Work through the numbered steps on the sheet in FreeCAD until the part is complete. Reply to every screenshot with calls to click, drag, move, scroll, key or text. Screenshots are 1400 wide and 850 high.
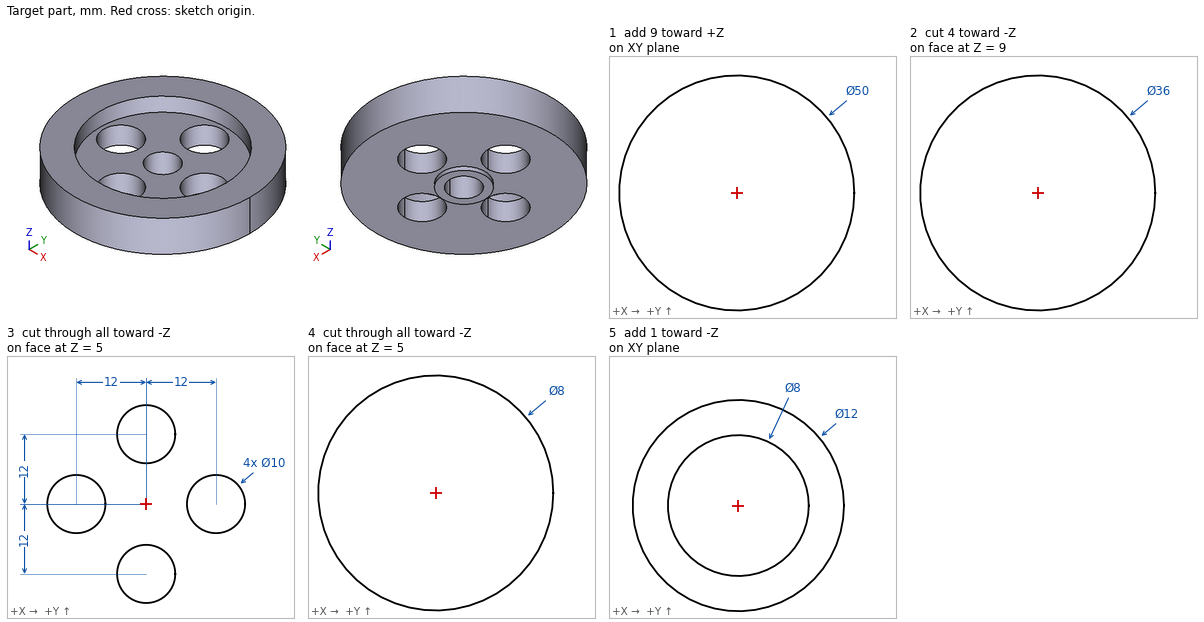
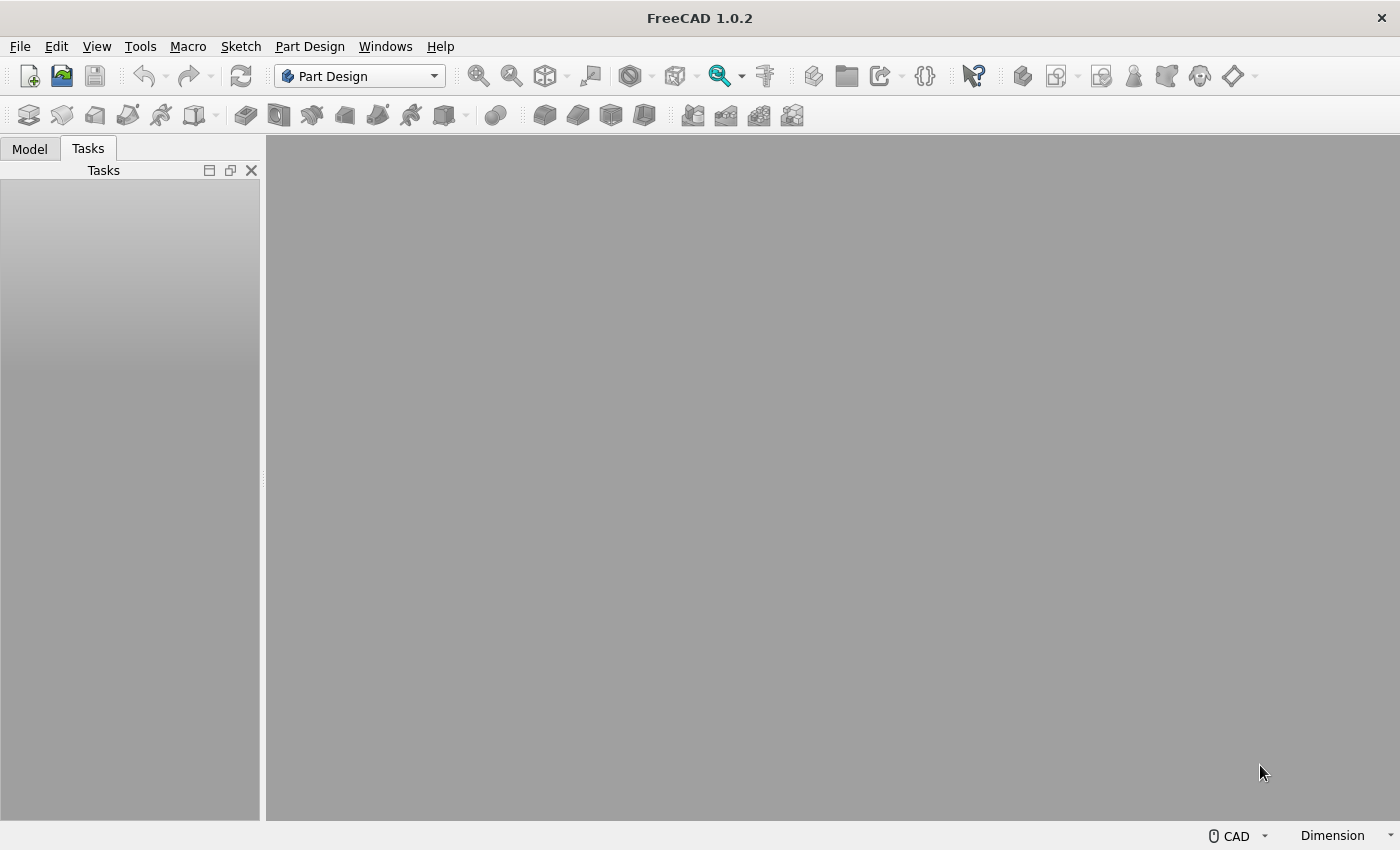
click(29, 76)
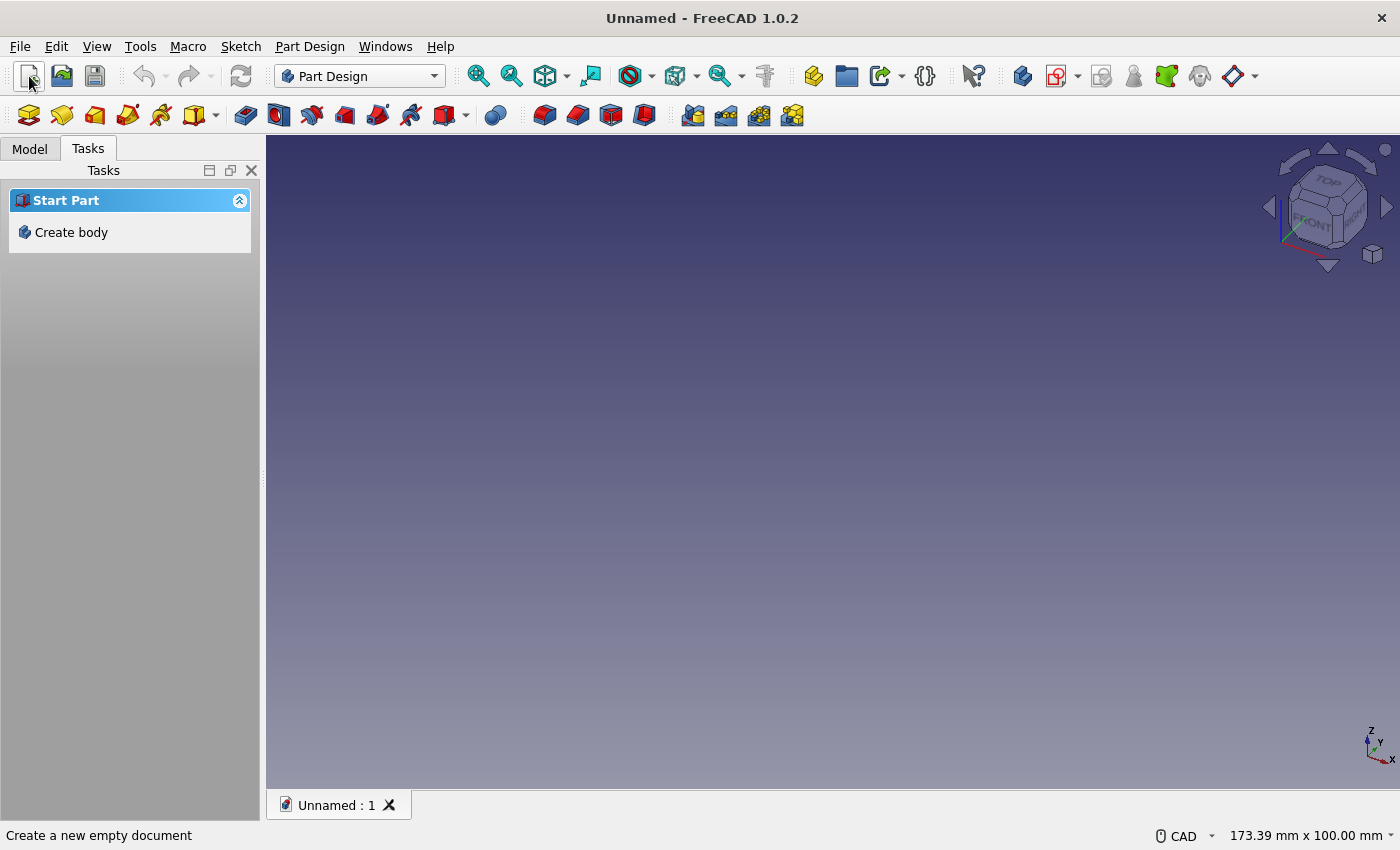
click(1056, 76)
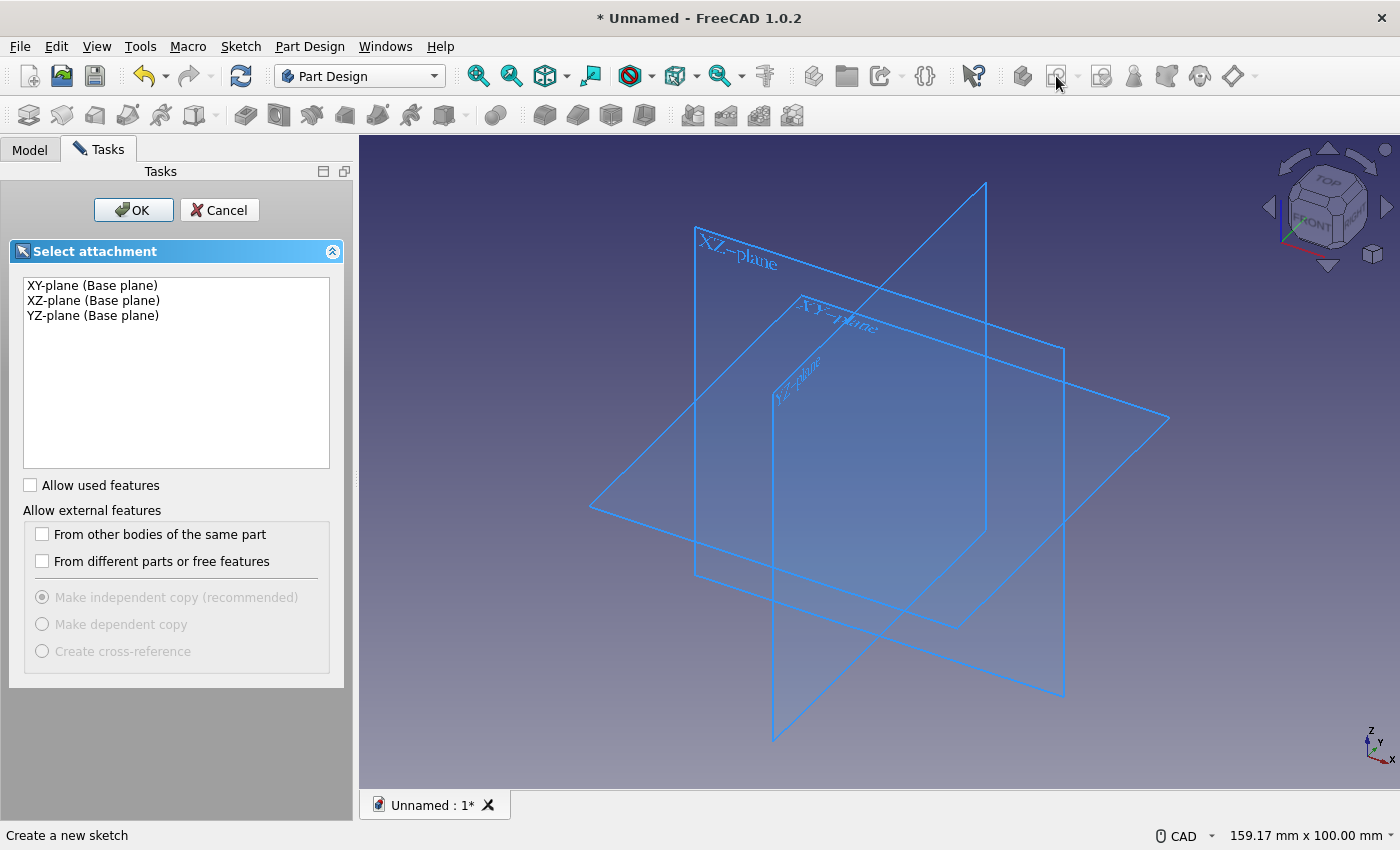
click(84, 286)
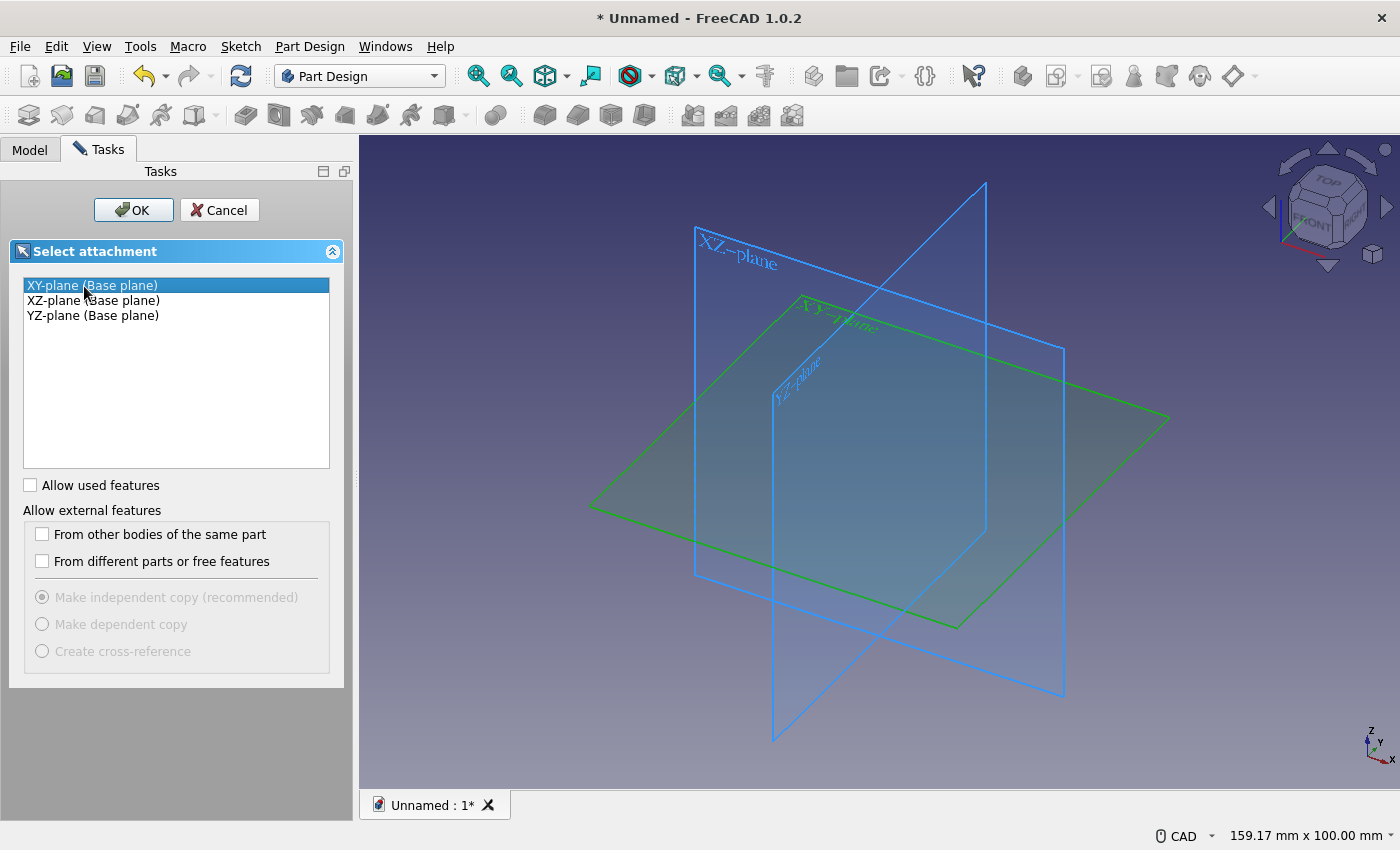
click(134, 210)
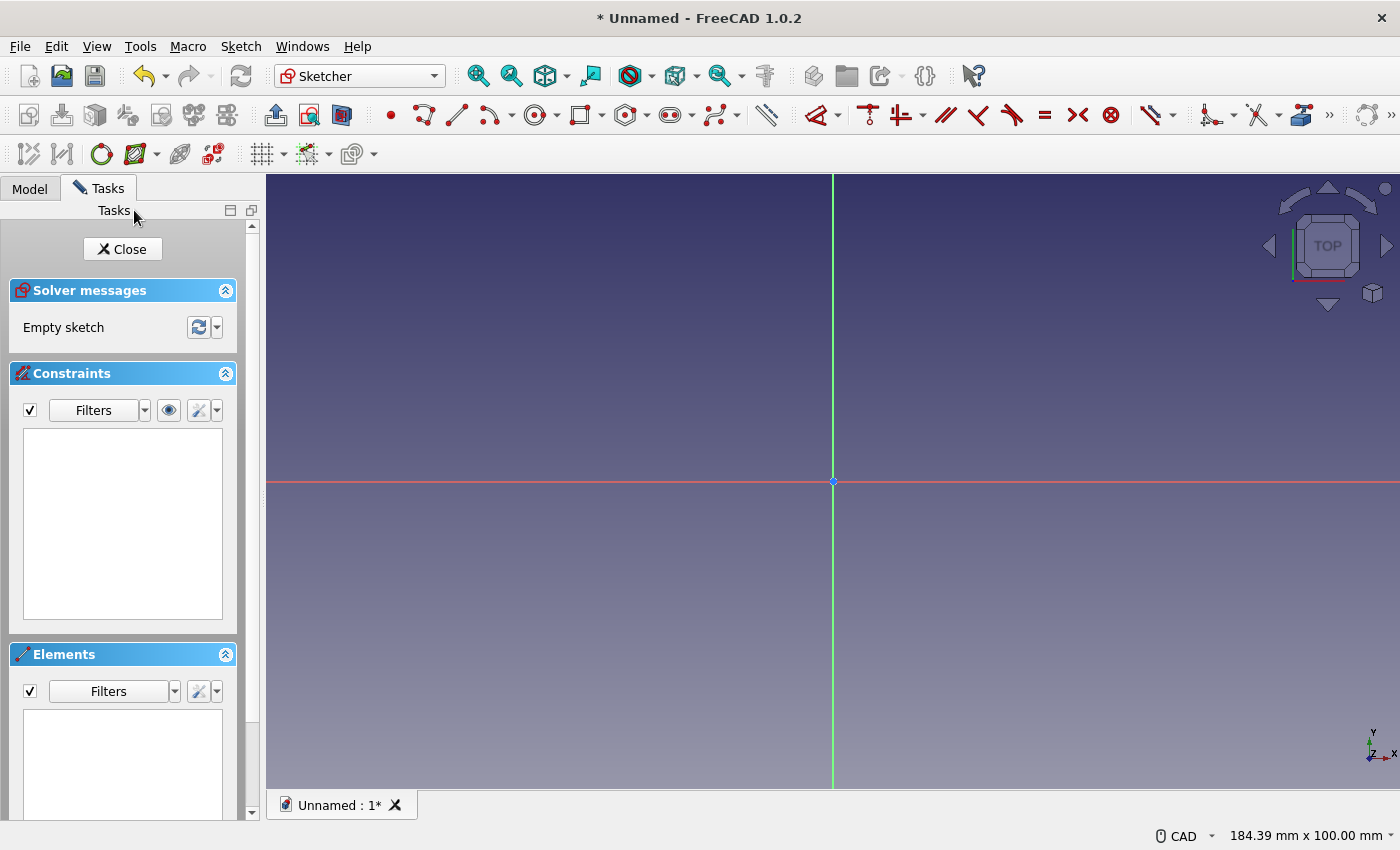
click(534, 116)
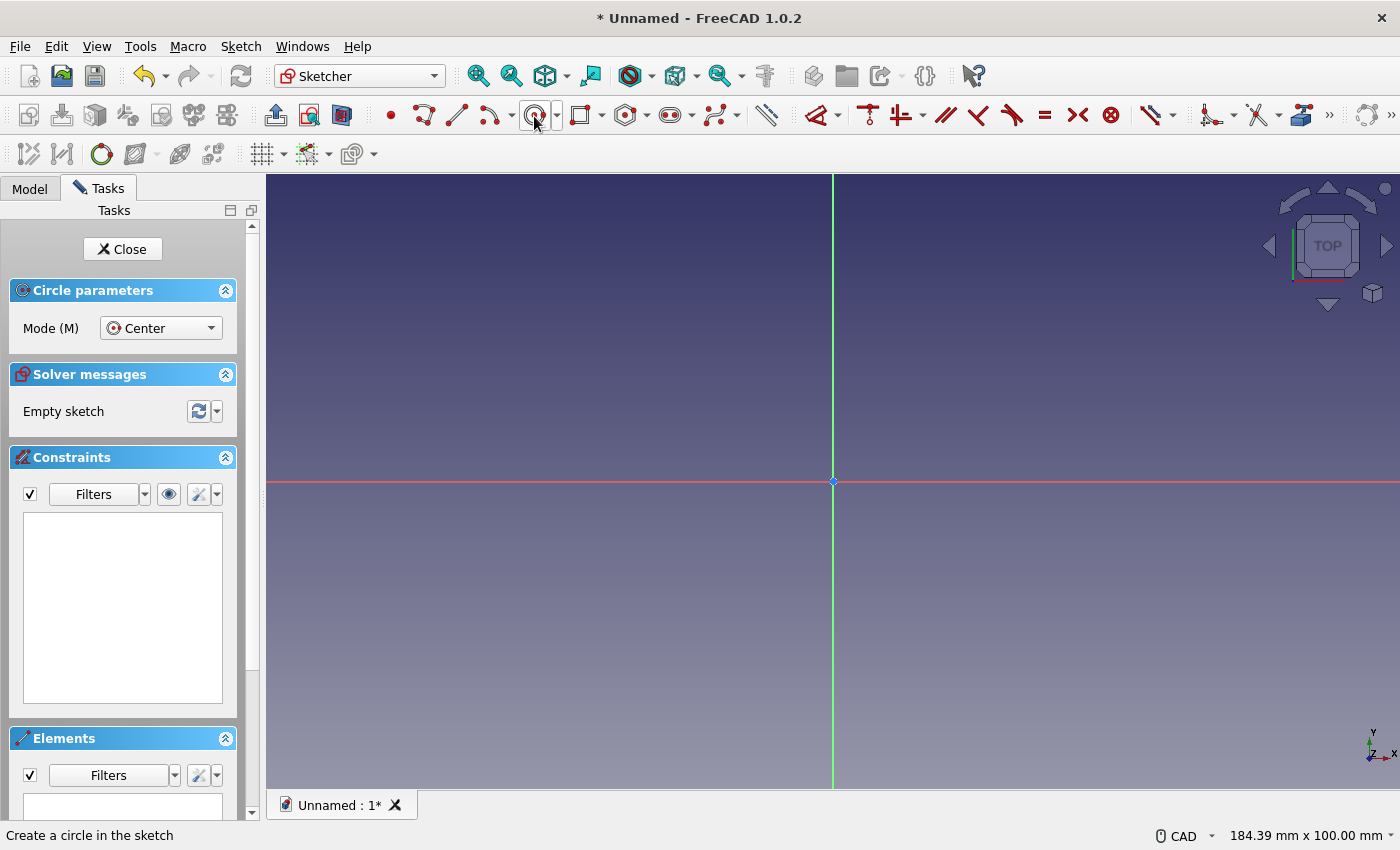
click(833, 482)
move(942, 373)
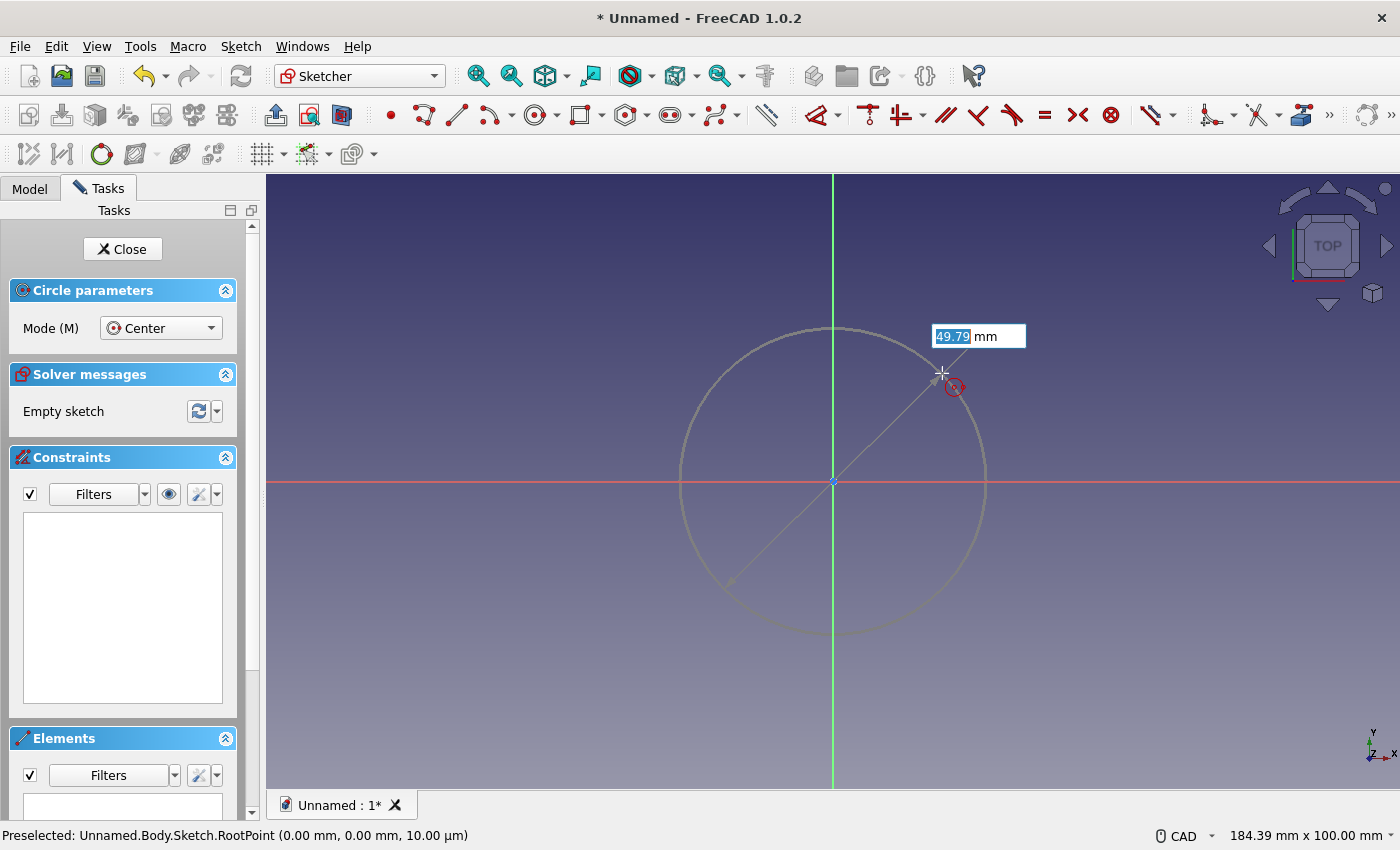
text(50)
key(Return)
key(Escape)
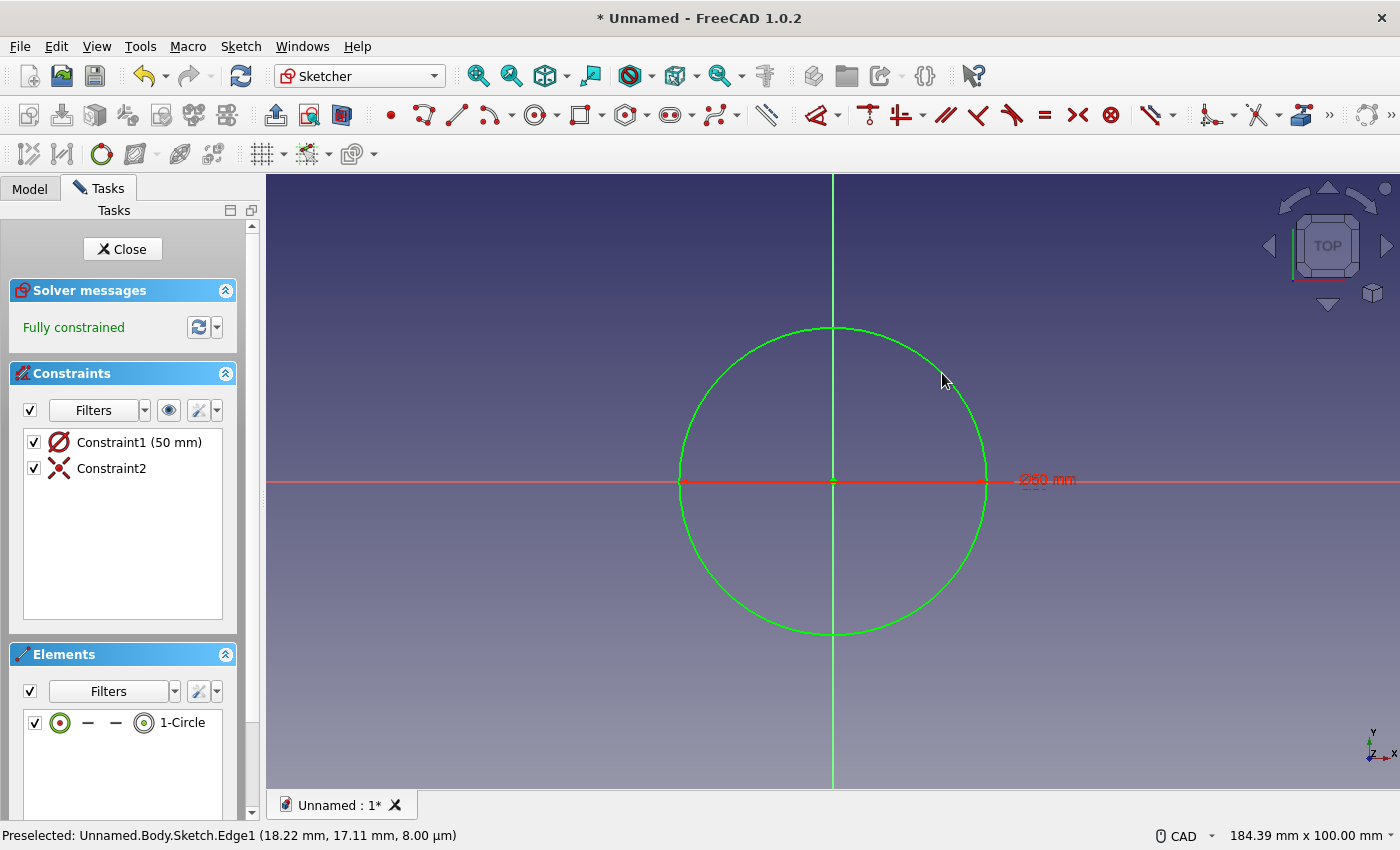
click(123, 249)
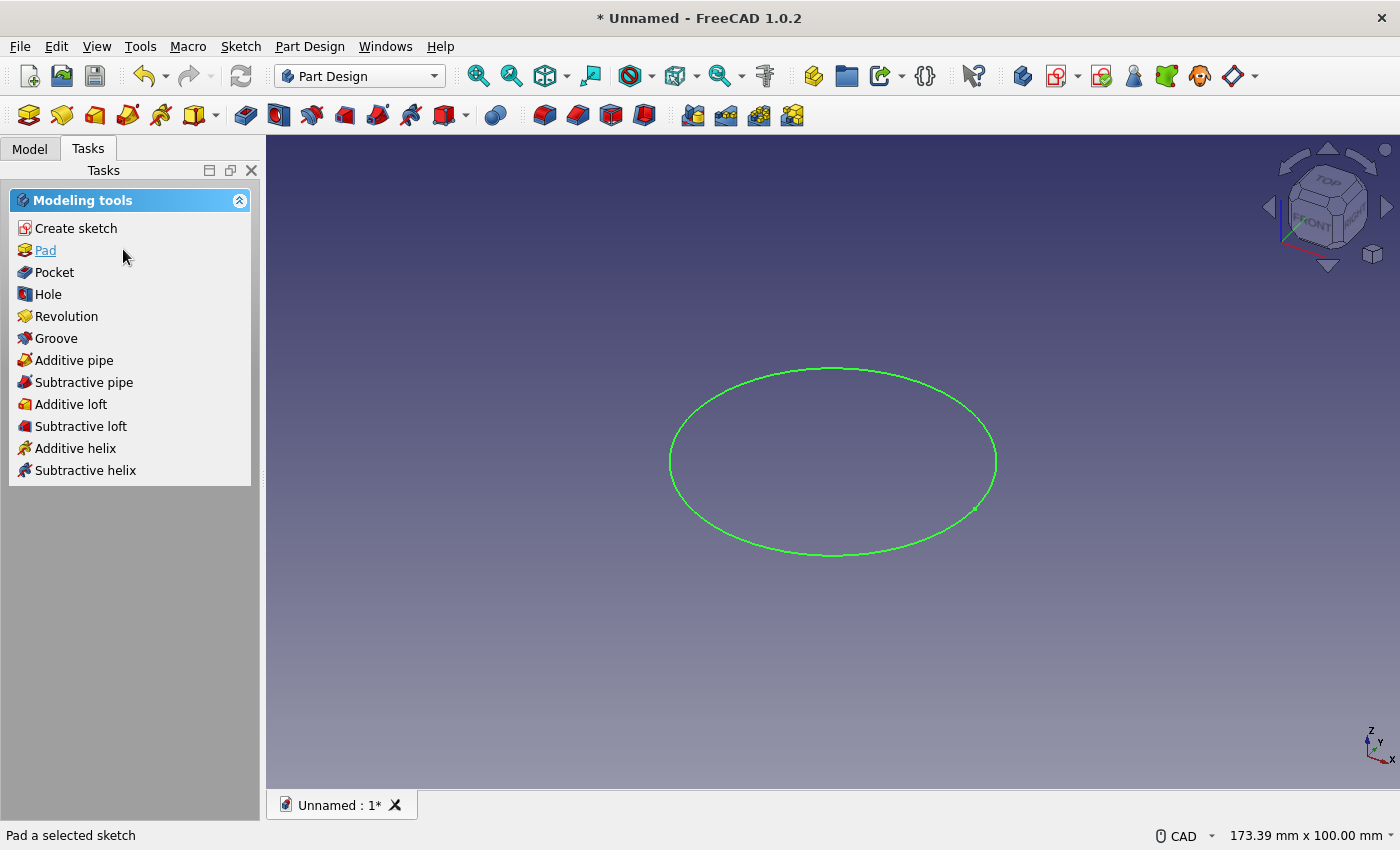
click(29, 116)